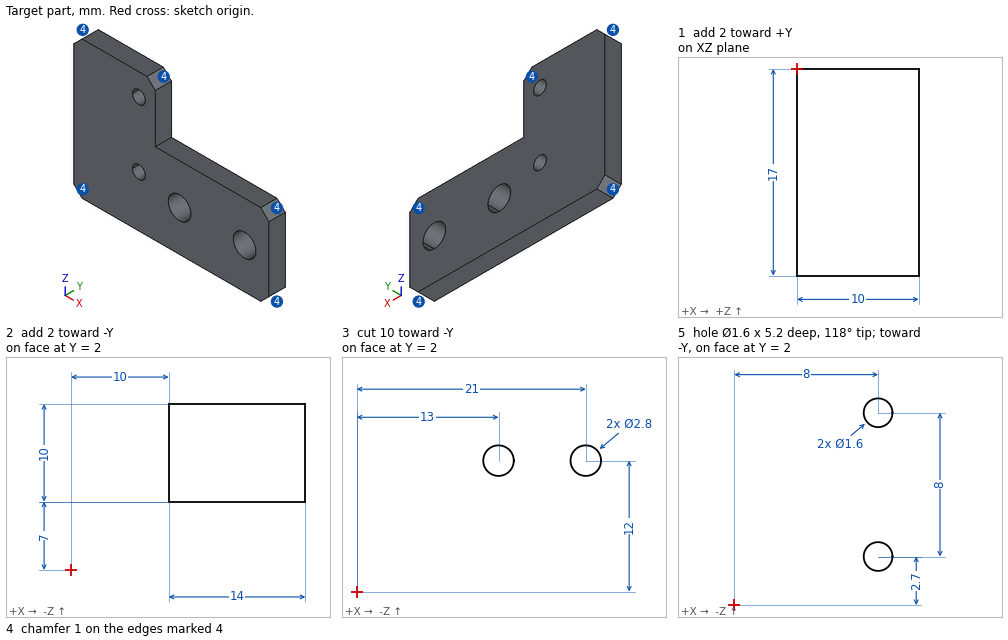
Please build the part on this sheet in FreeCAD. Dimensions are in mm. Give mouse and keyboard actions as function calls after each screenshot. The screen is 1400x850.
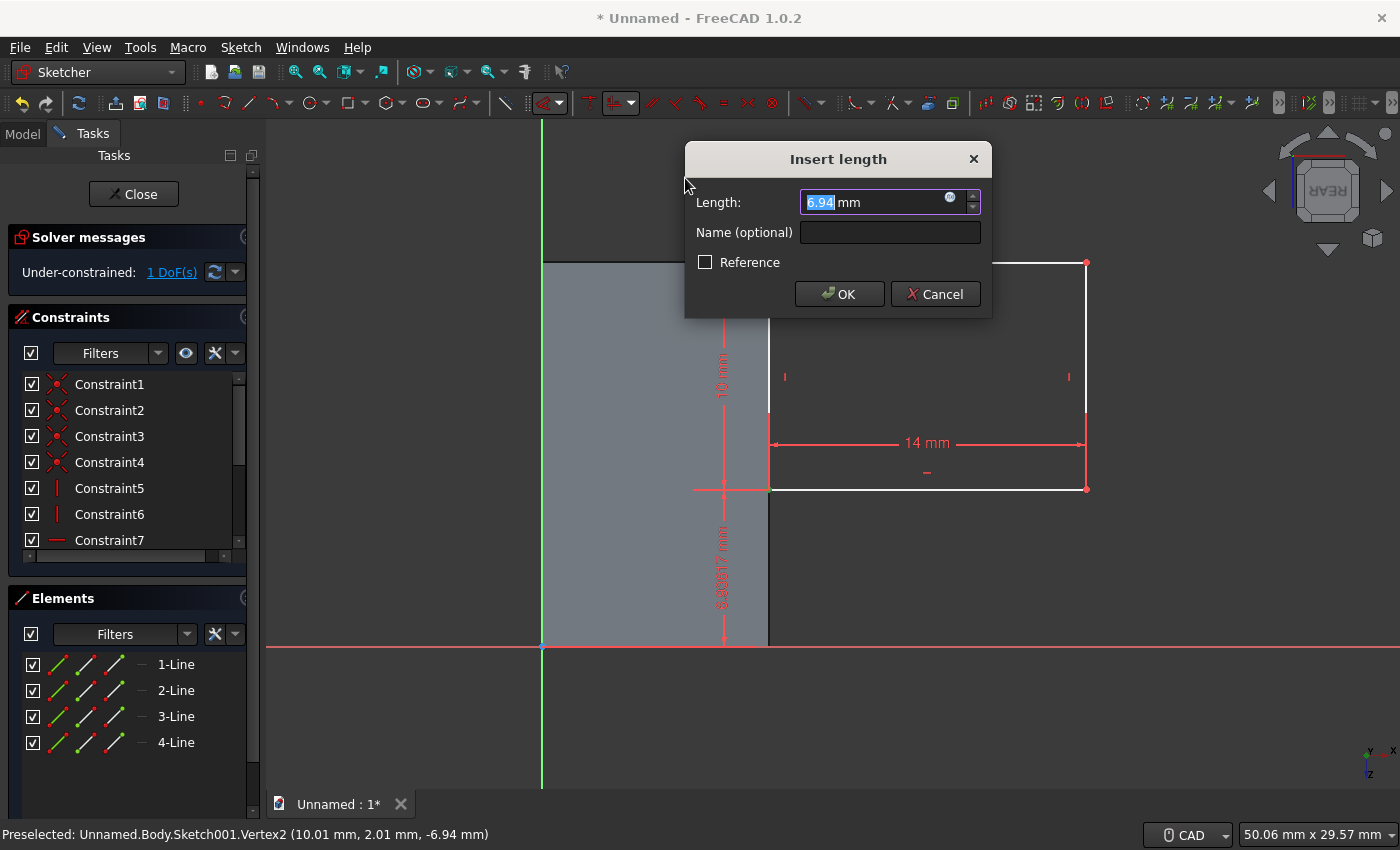
text(7)
key(Return)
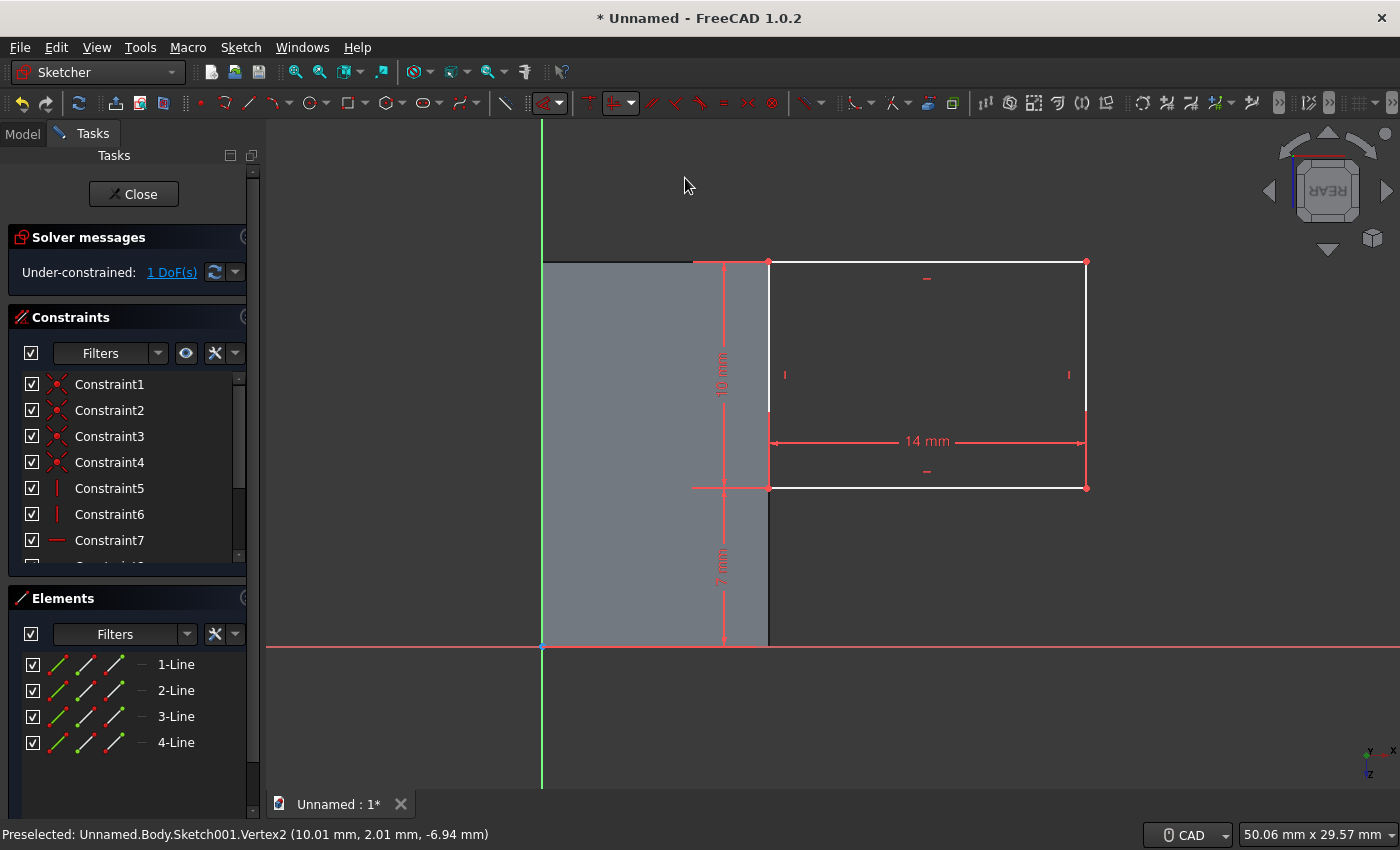
click(769, 262)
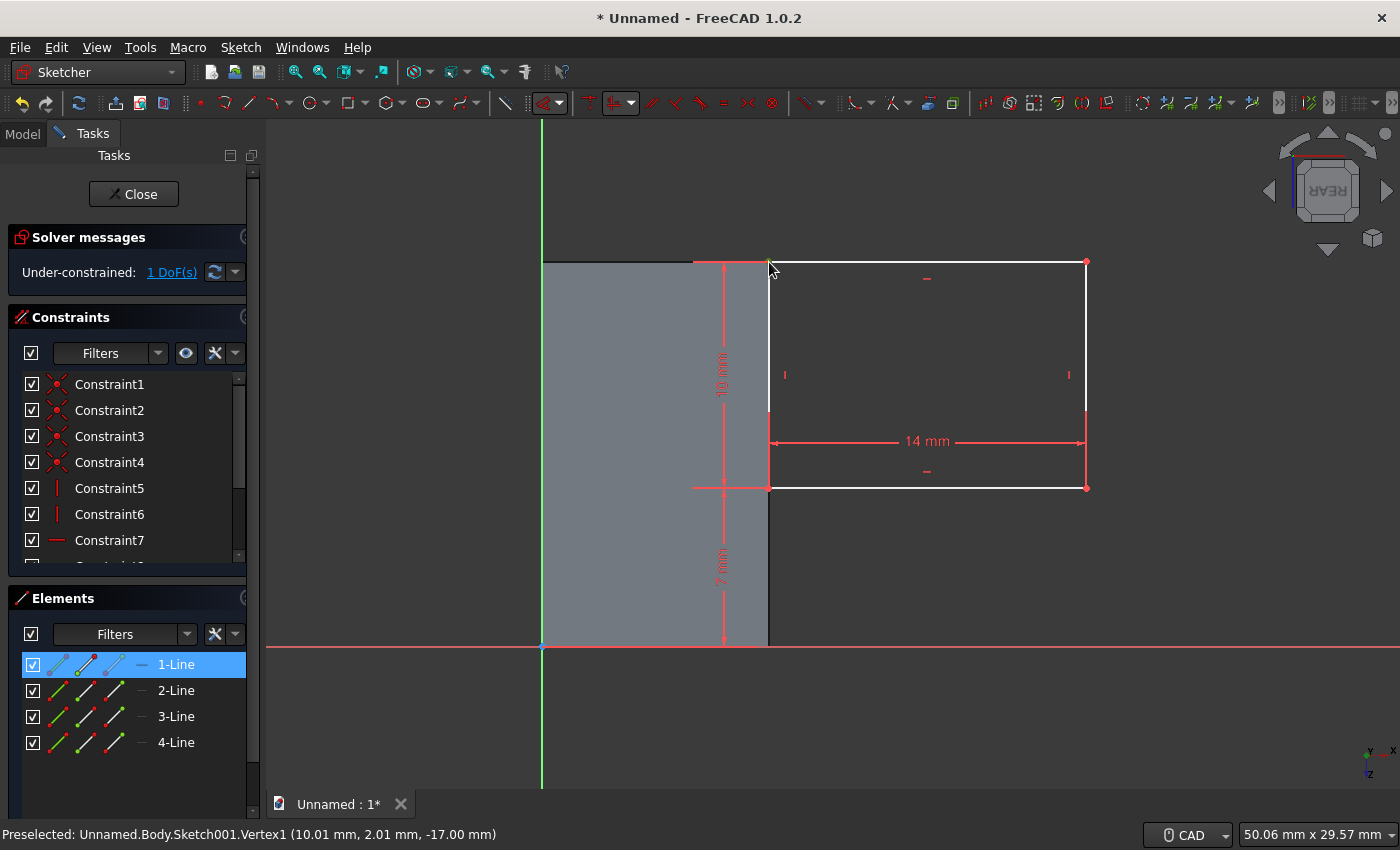
click(562, 104)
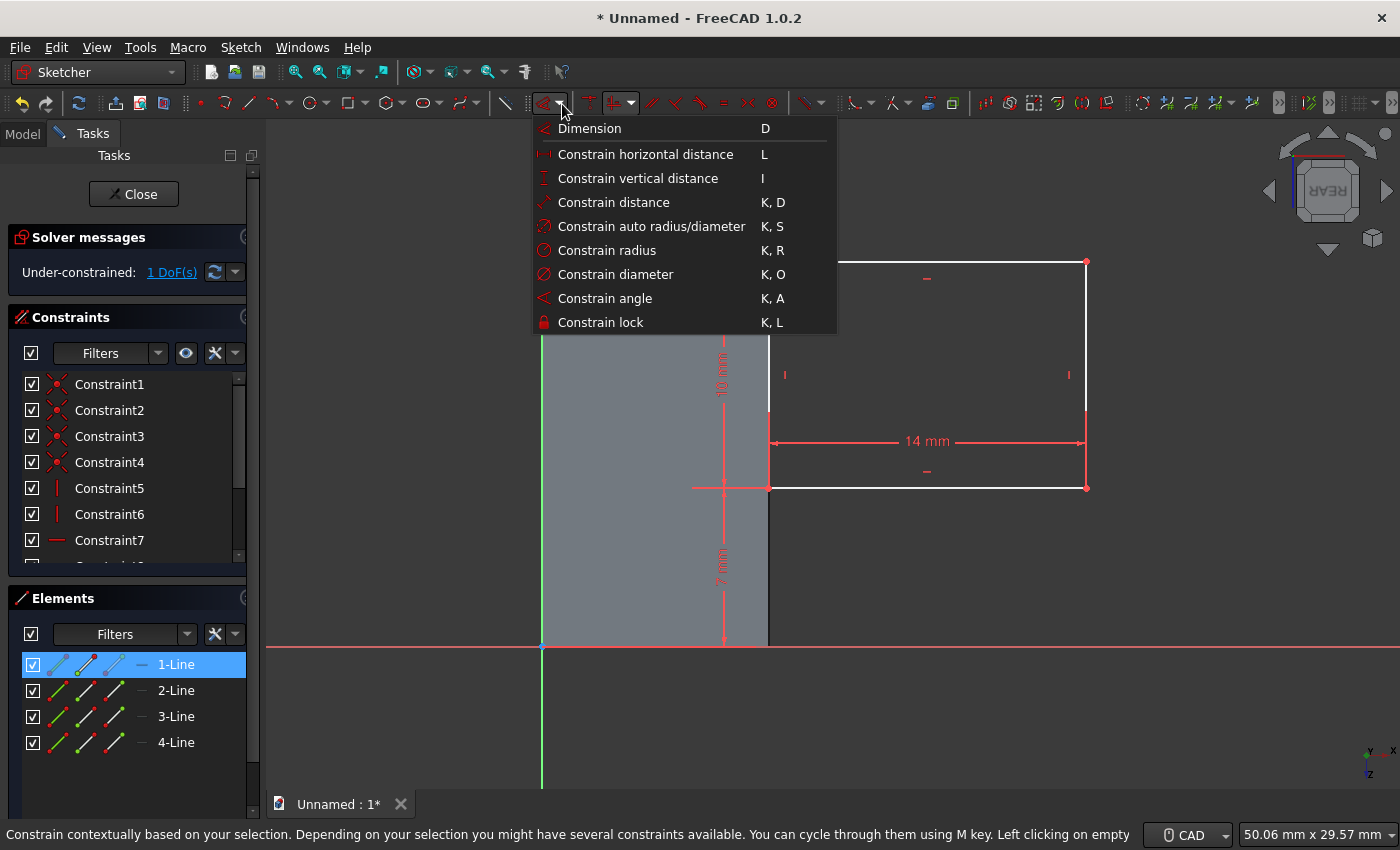
click(685, 154)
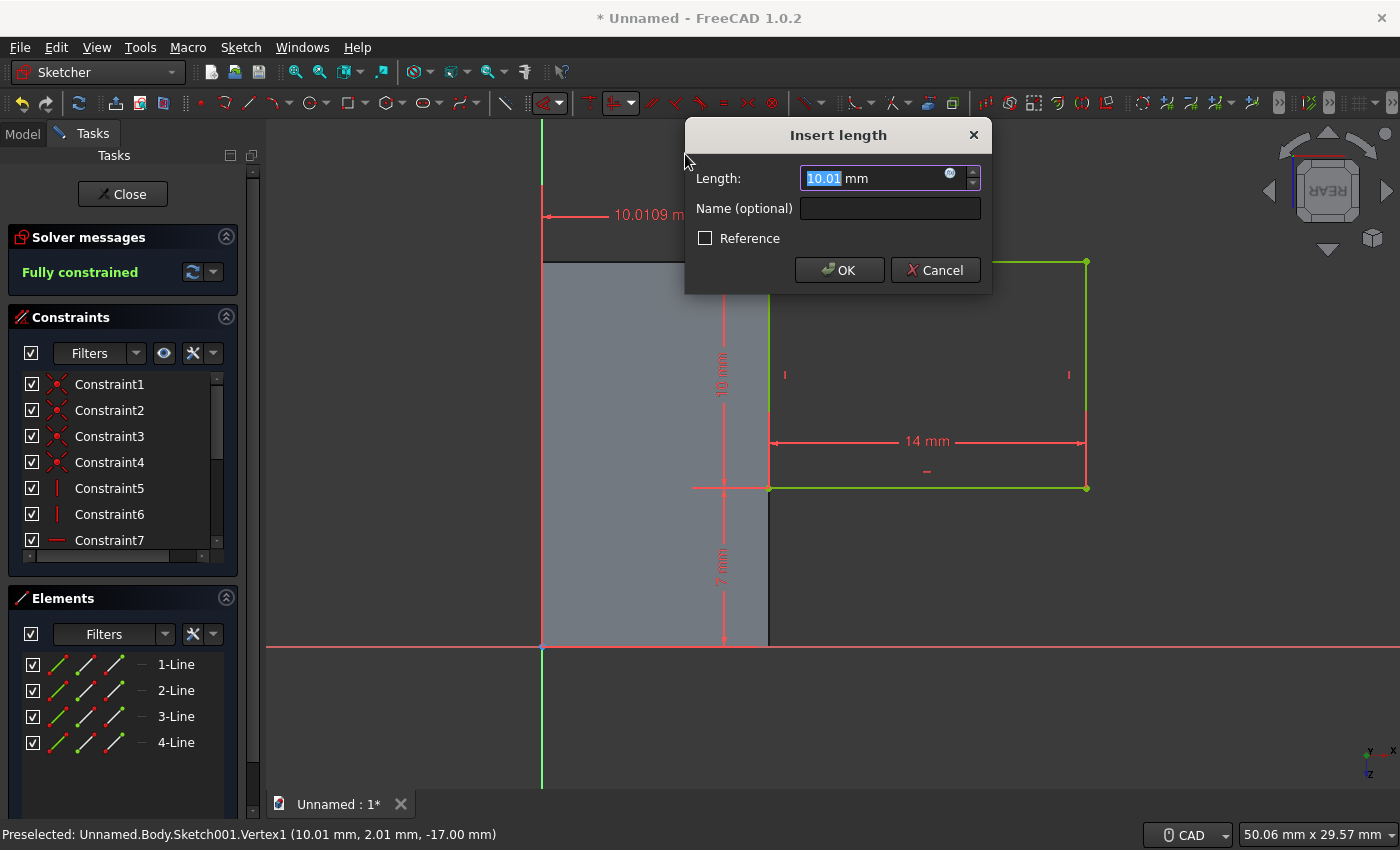
text(10)
key(Return)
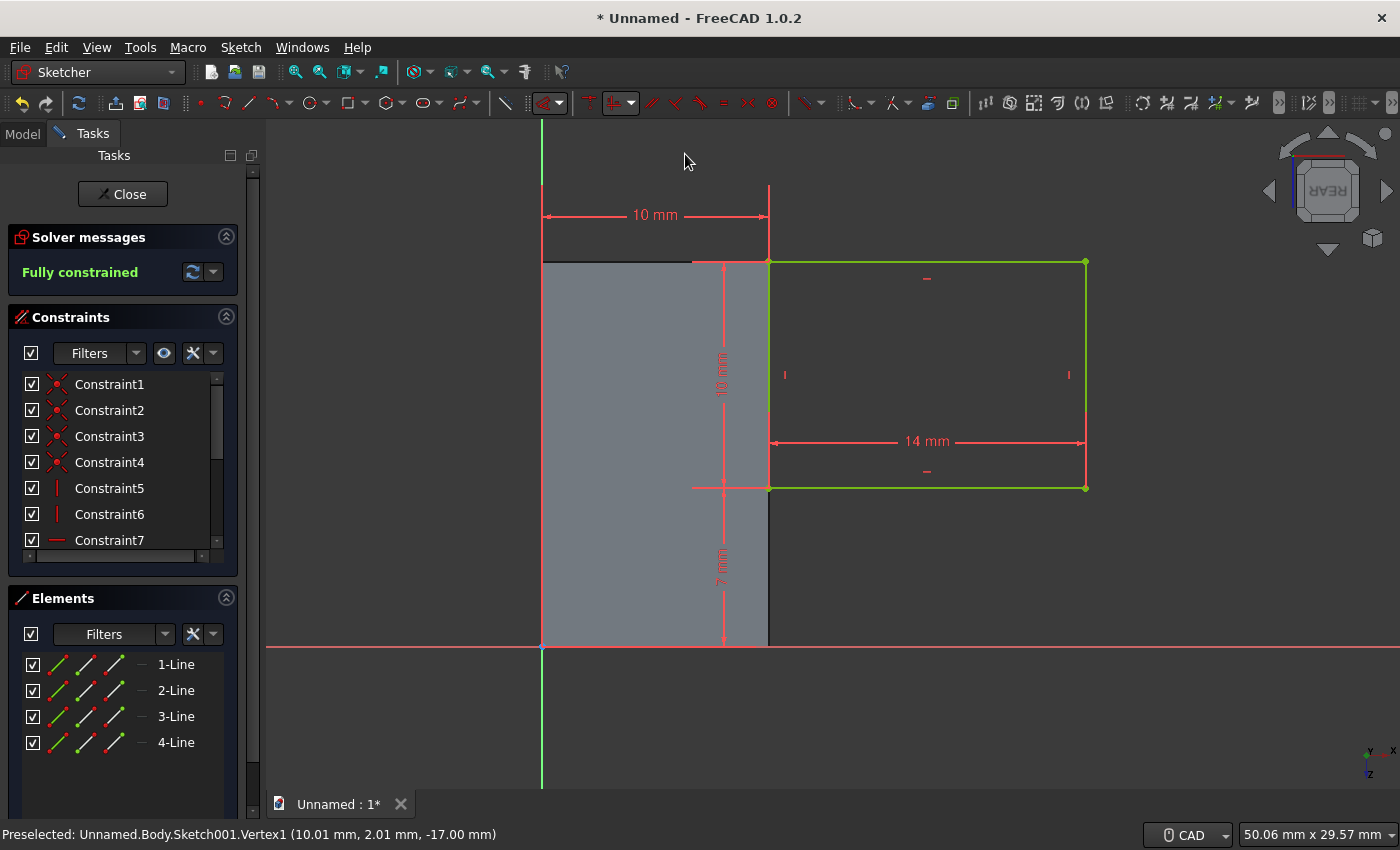
click(123, 194)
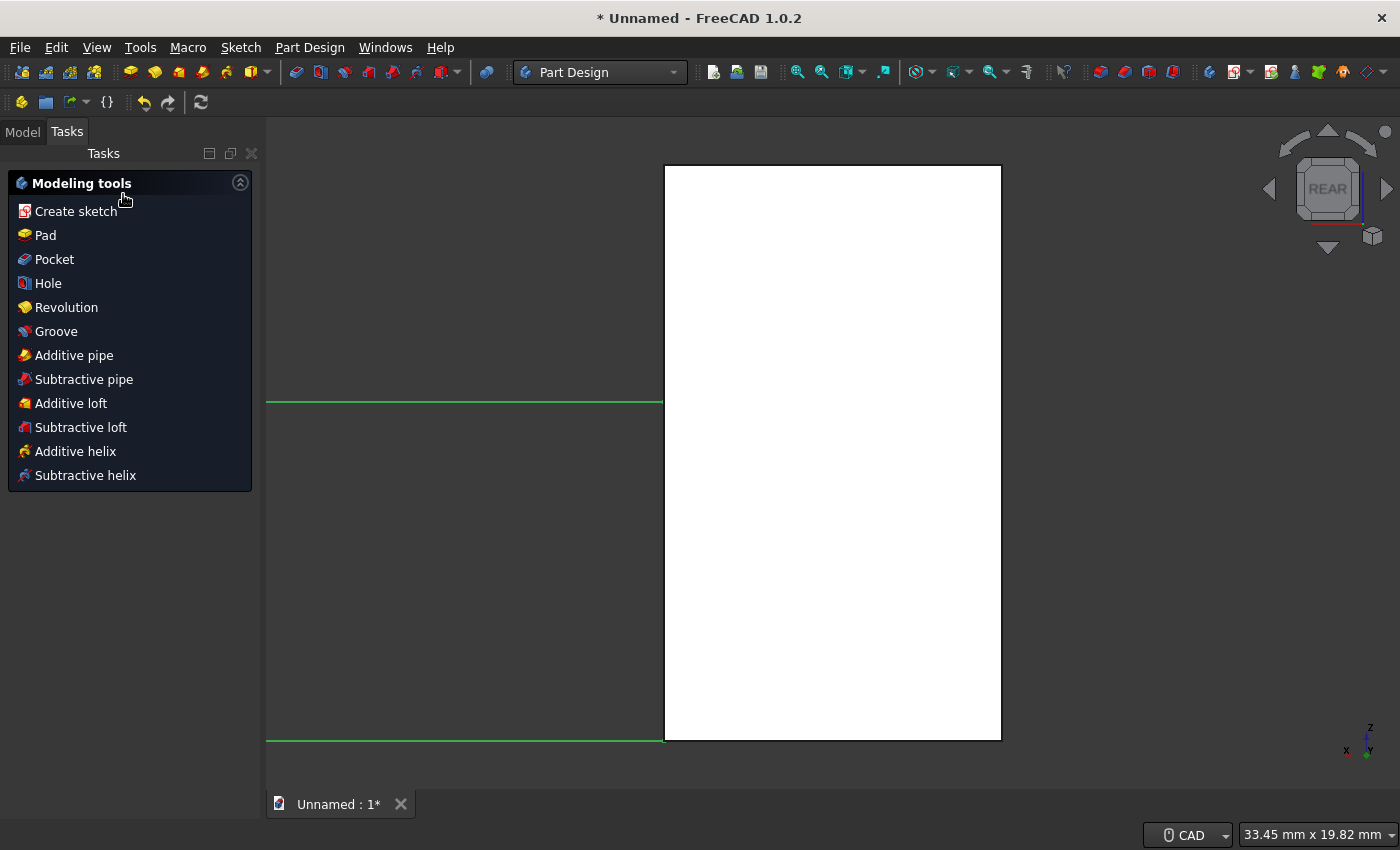
click(132, 72)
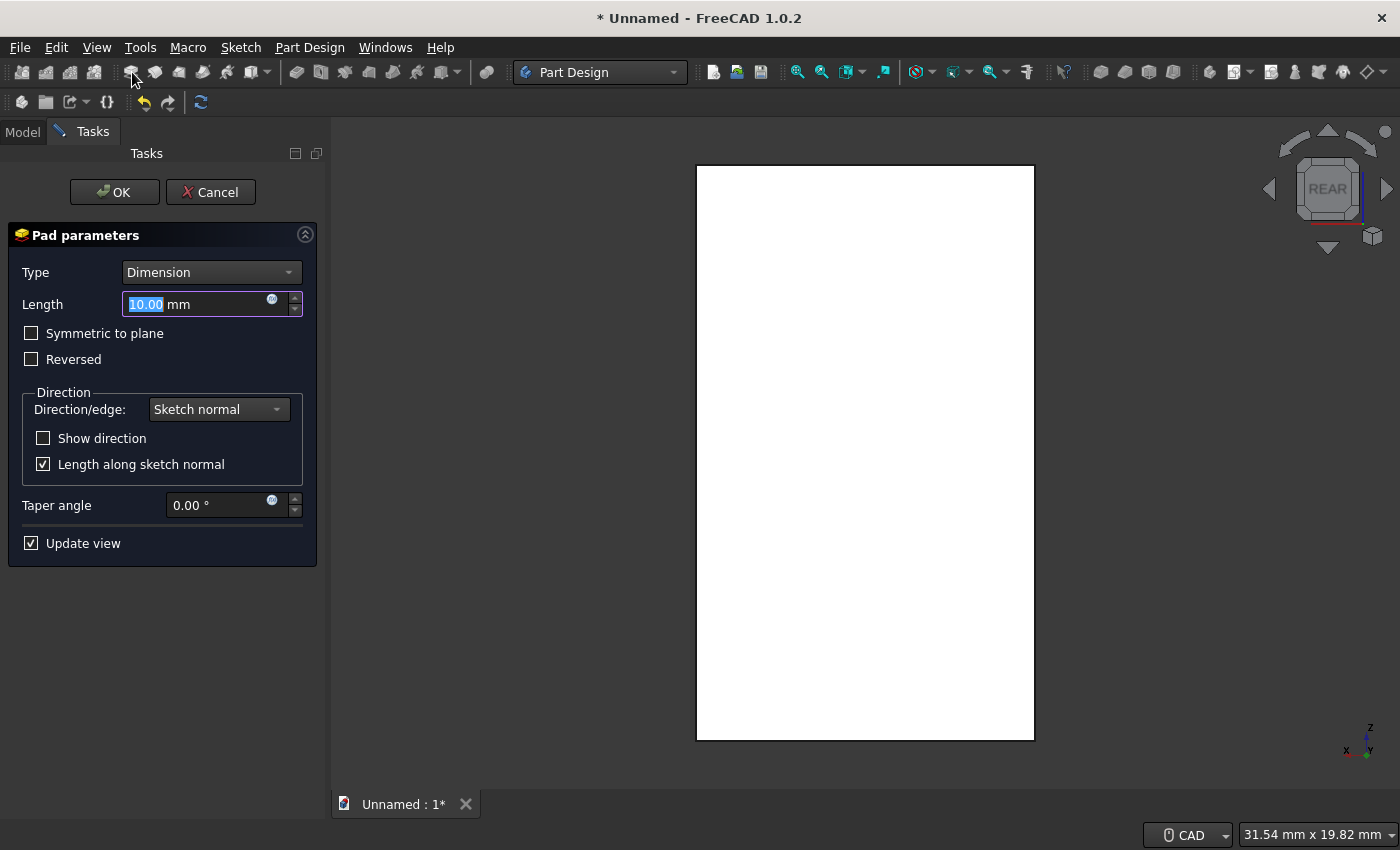
text(2)
key(Tab)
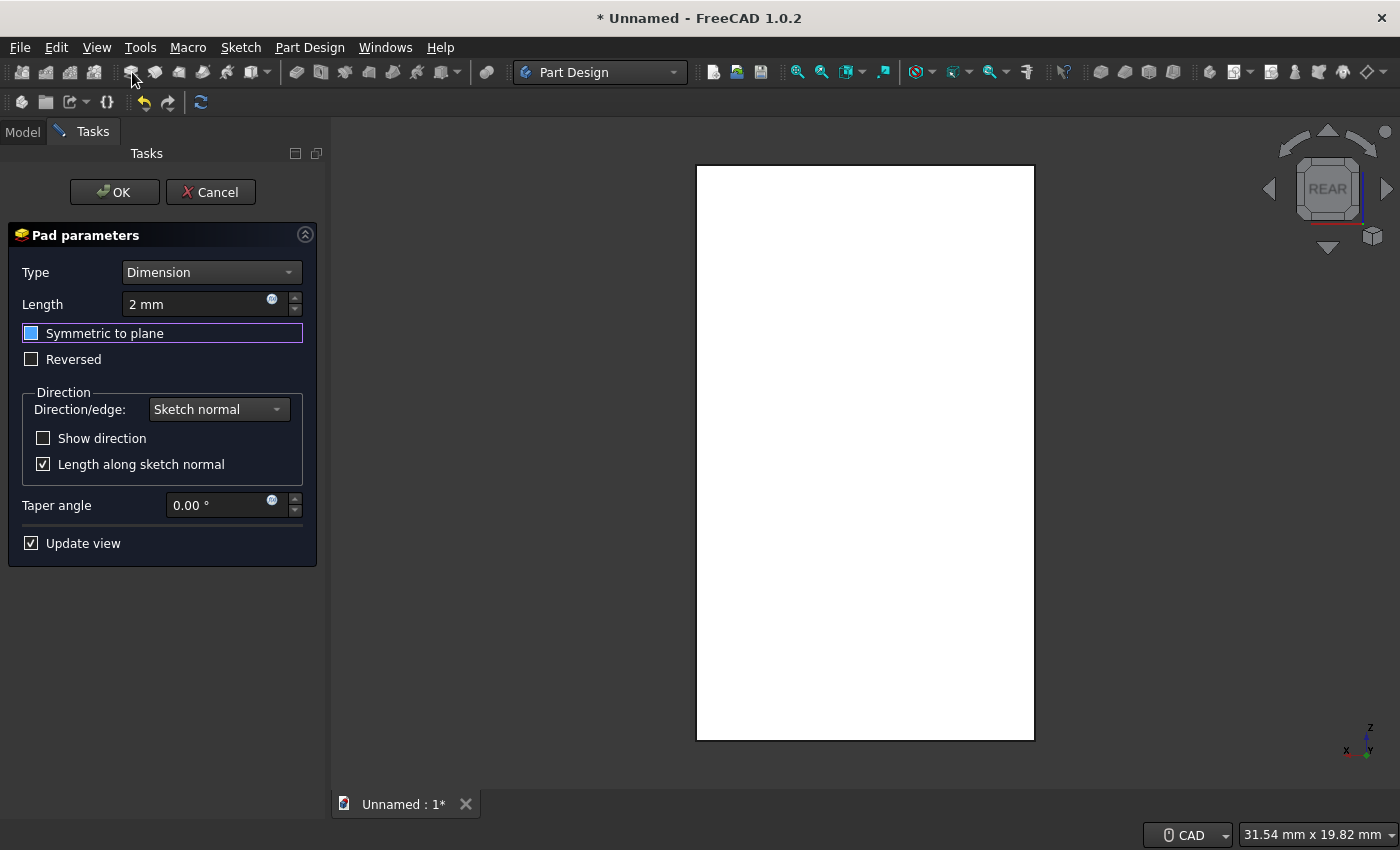
click(30, 359)